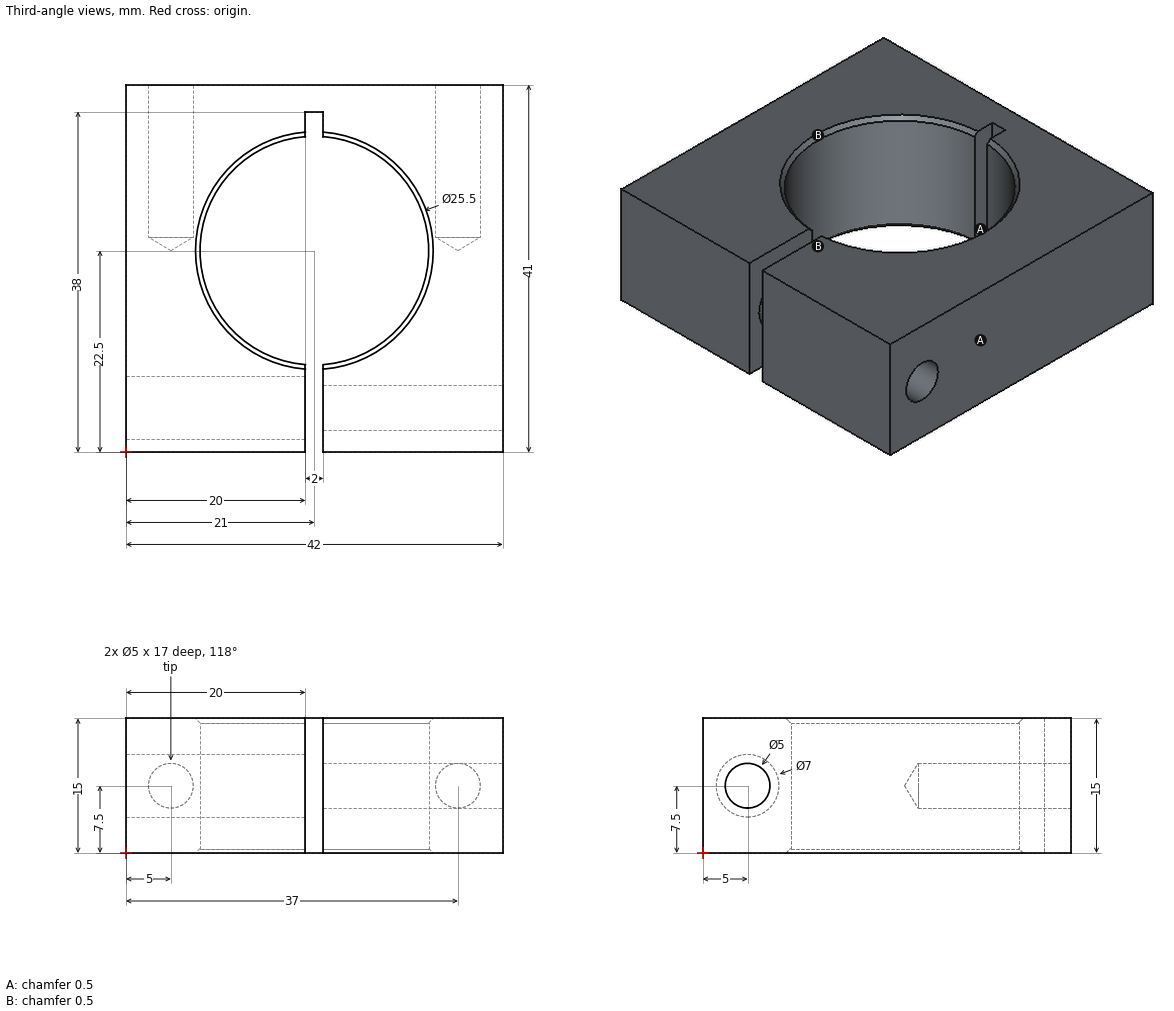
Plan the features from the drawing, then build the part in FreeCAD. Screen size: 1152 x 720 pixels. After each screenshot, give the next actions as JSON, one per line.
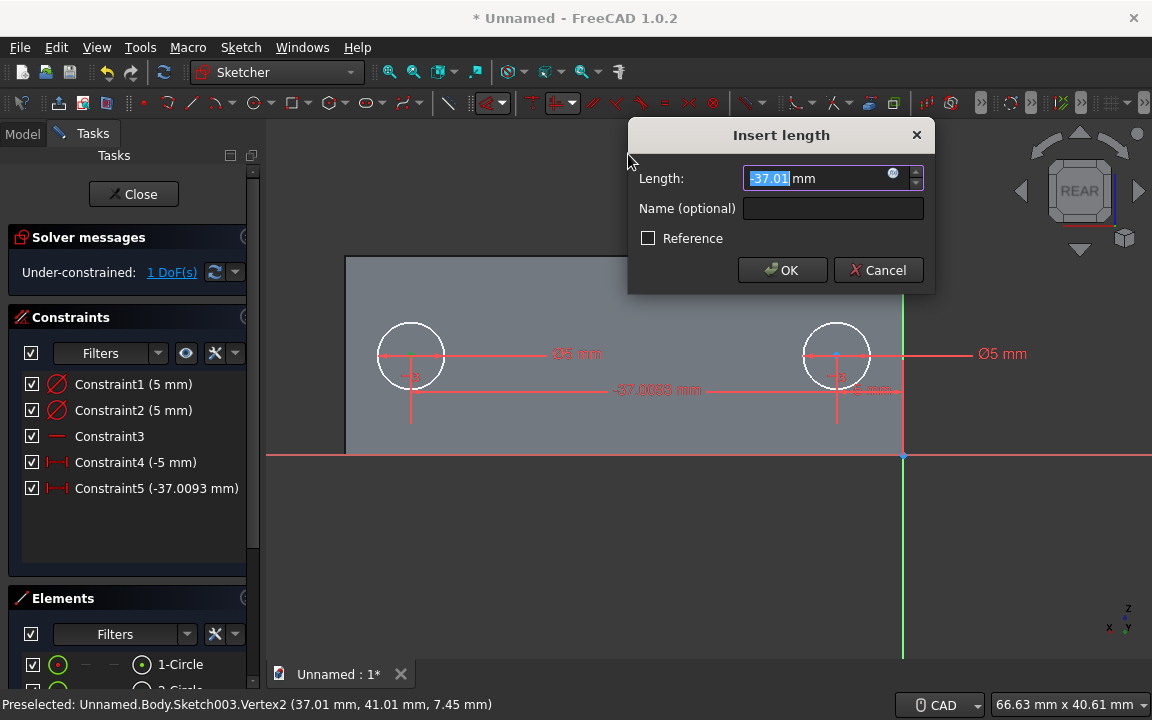
{"action": "type", "text": "-37"}
{"action": "key", "text": "Return"}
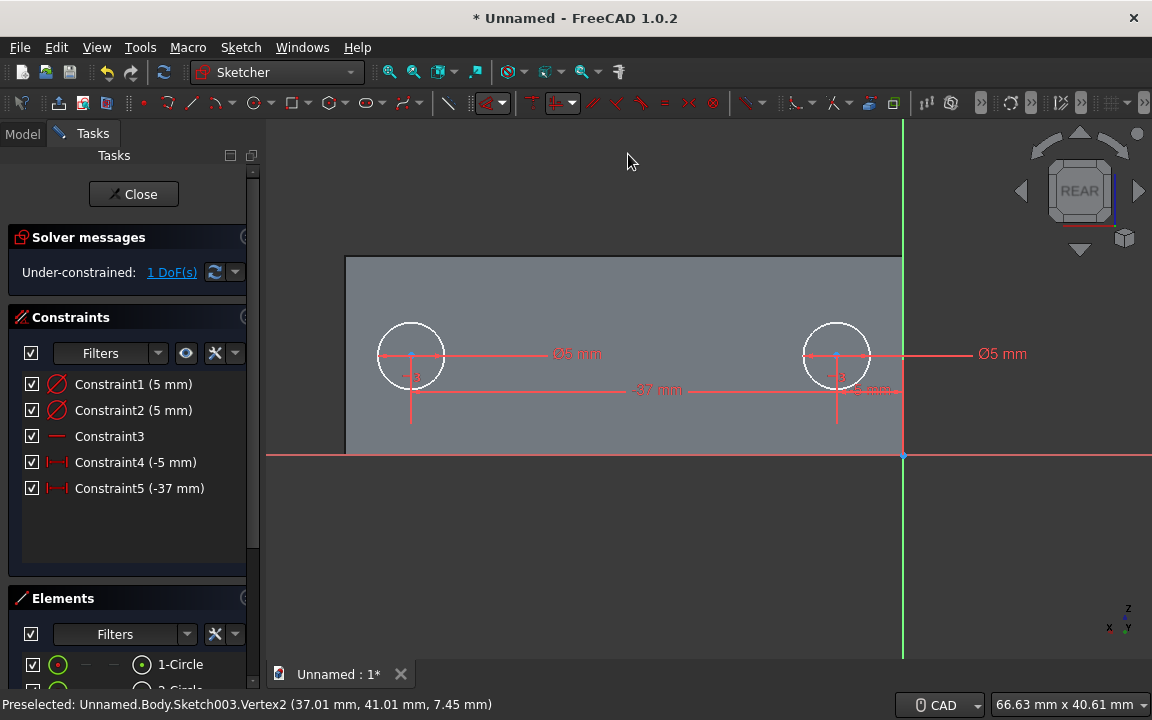
{"action": "left_click", "coordinate": [837, 356]}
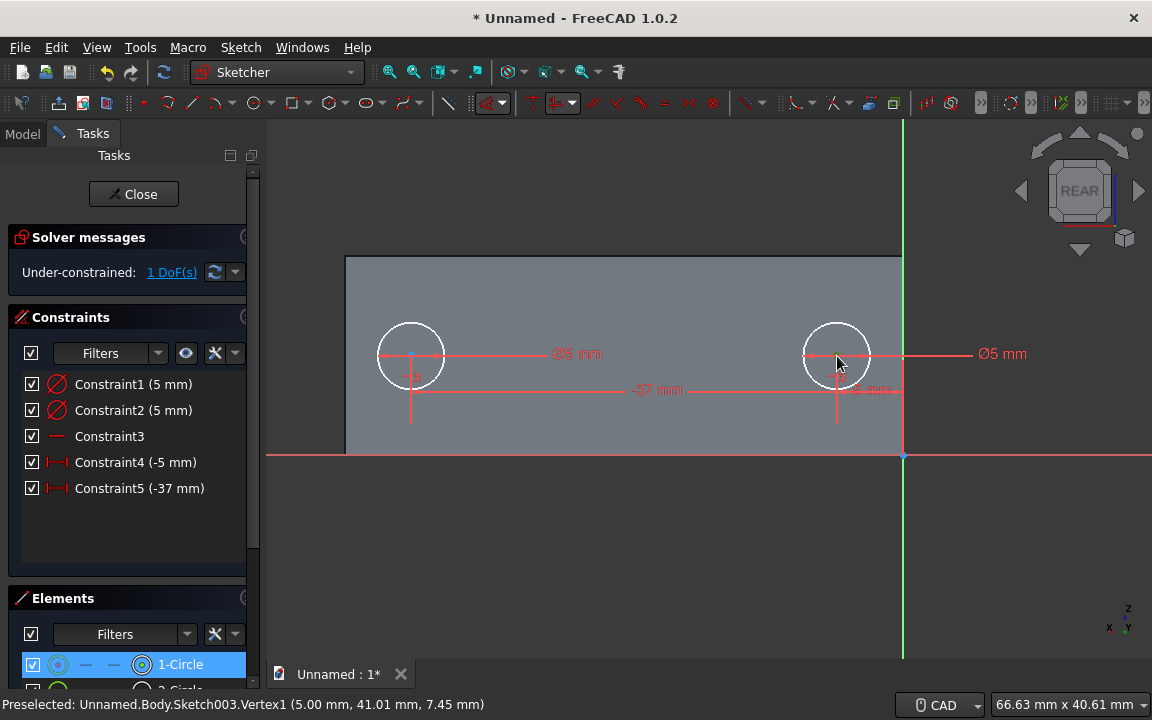
{"action": "left_click", "coordinate": [504, 104]}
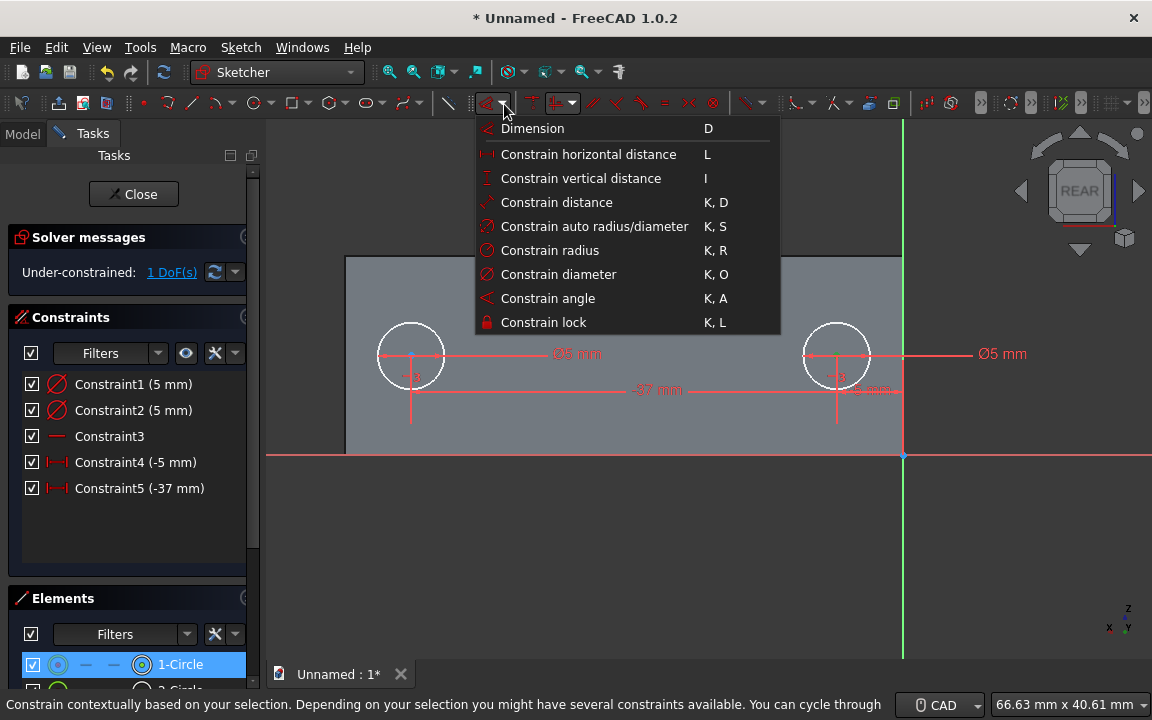
{"action": "left_click", "coordinate": [628, 178]}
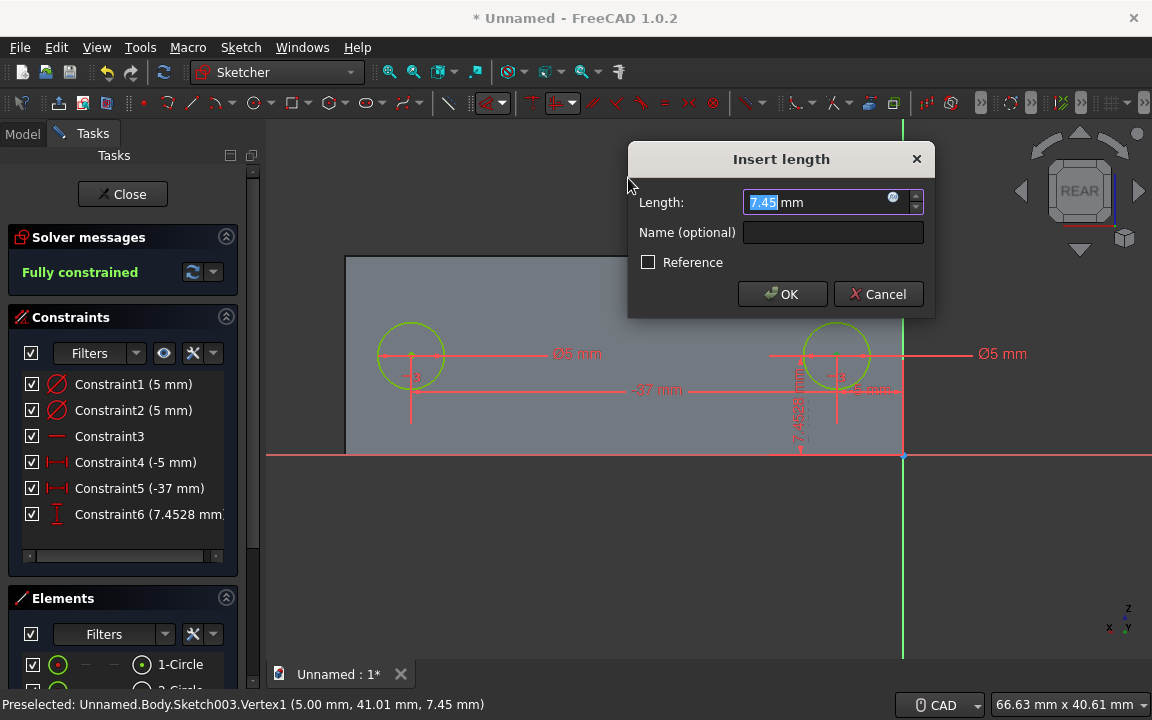
{"action": "type", "text": "7.5"}
{"action": "key", "text": "Return"}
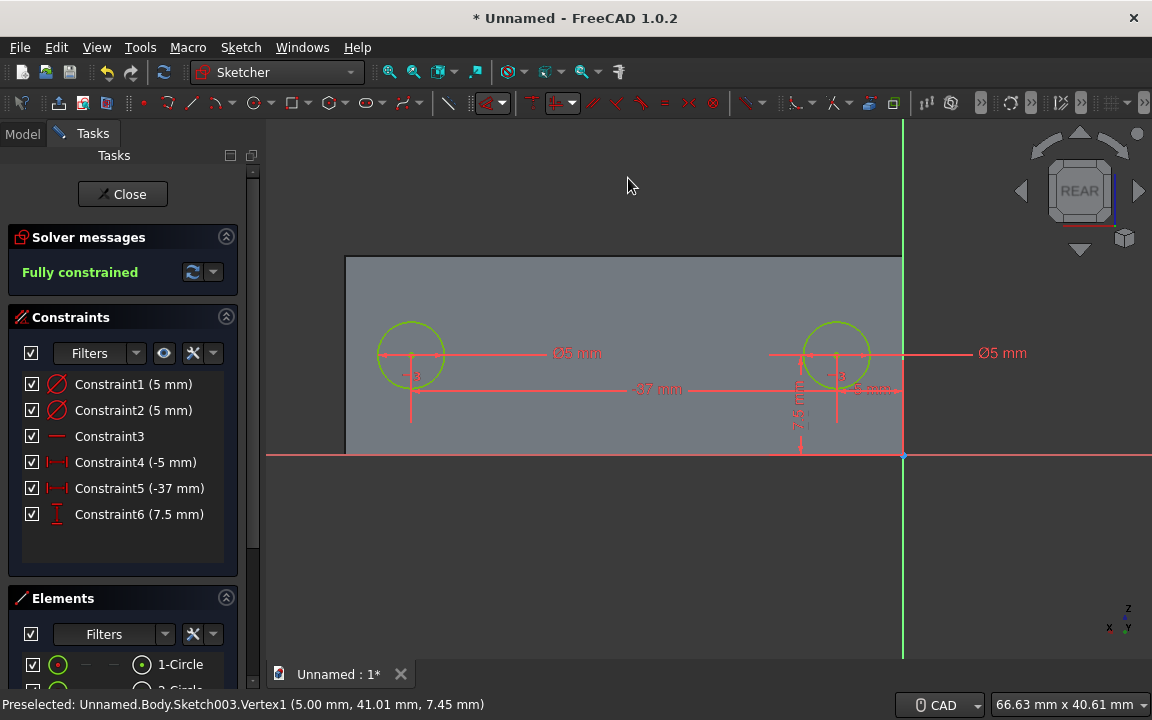
{"action": "left_click", "coordinate": [123, 194]}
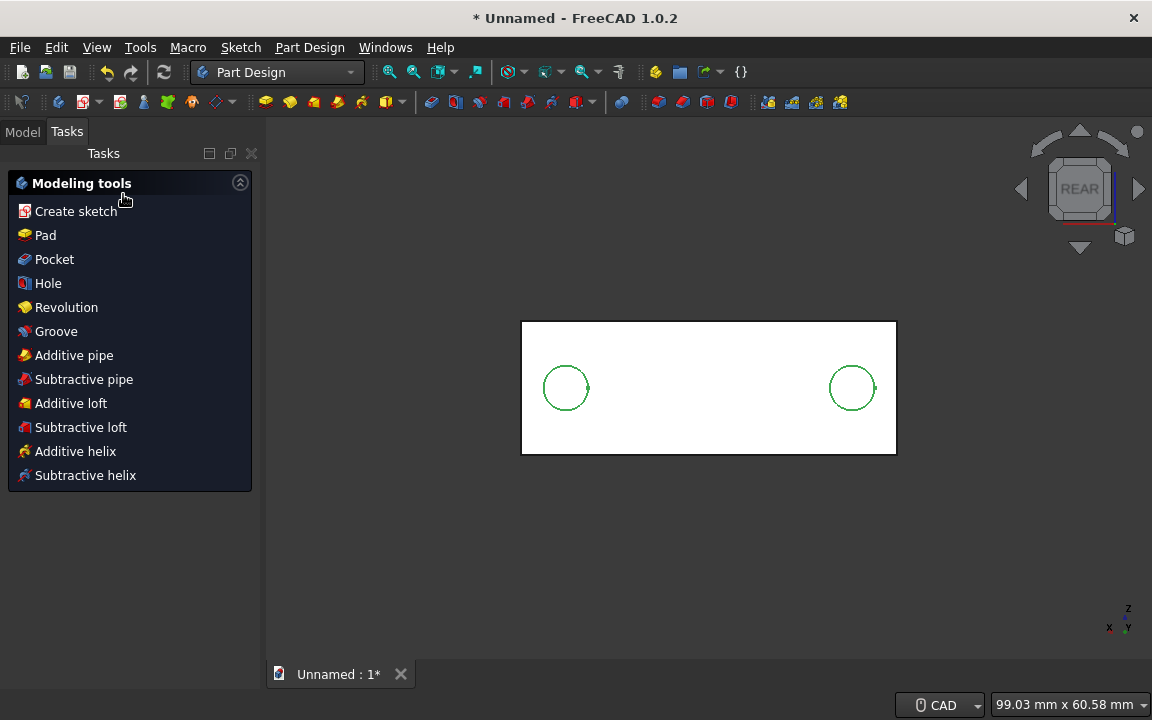
{"action": "left_click", "coordinate": [456, 102]}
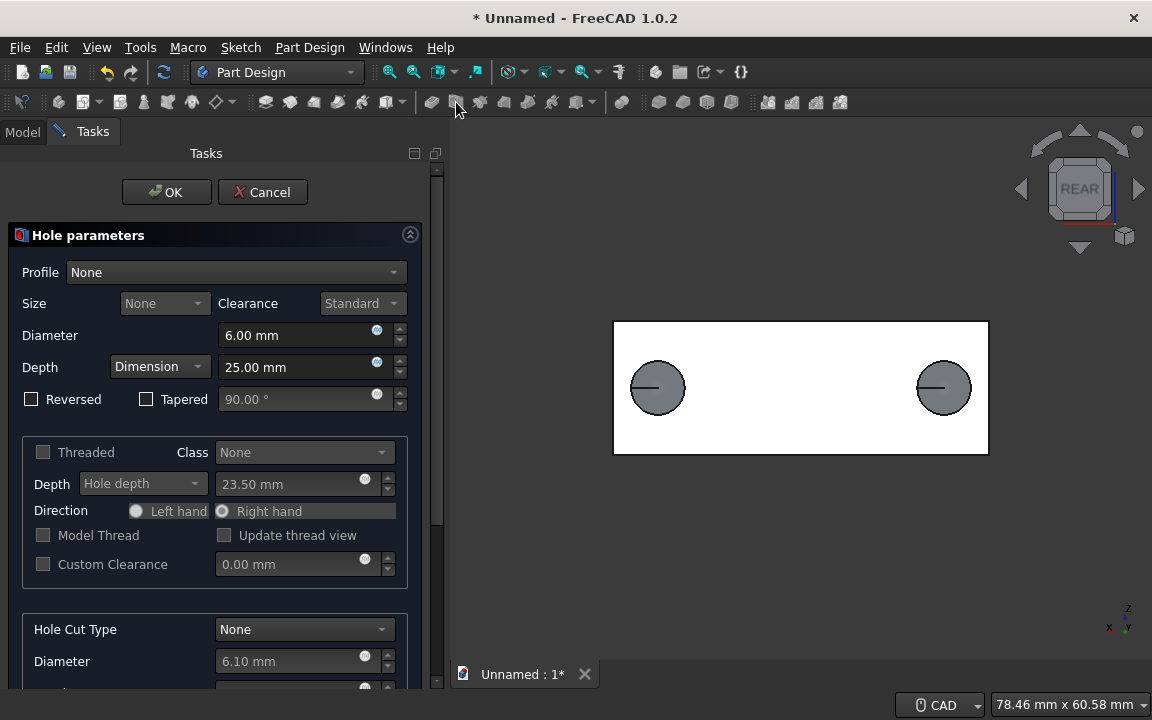
{"action": "triple_click", "coordinate": [305, 335]}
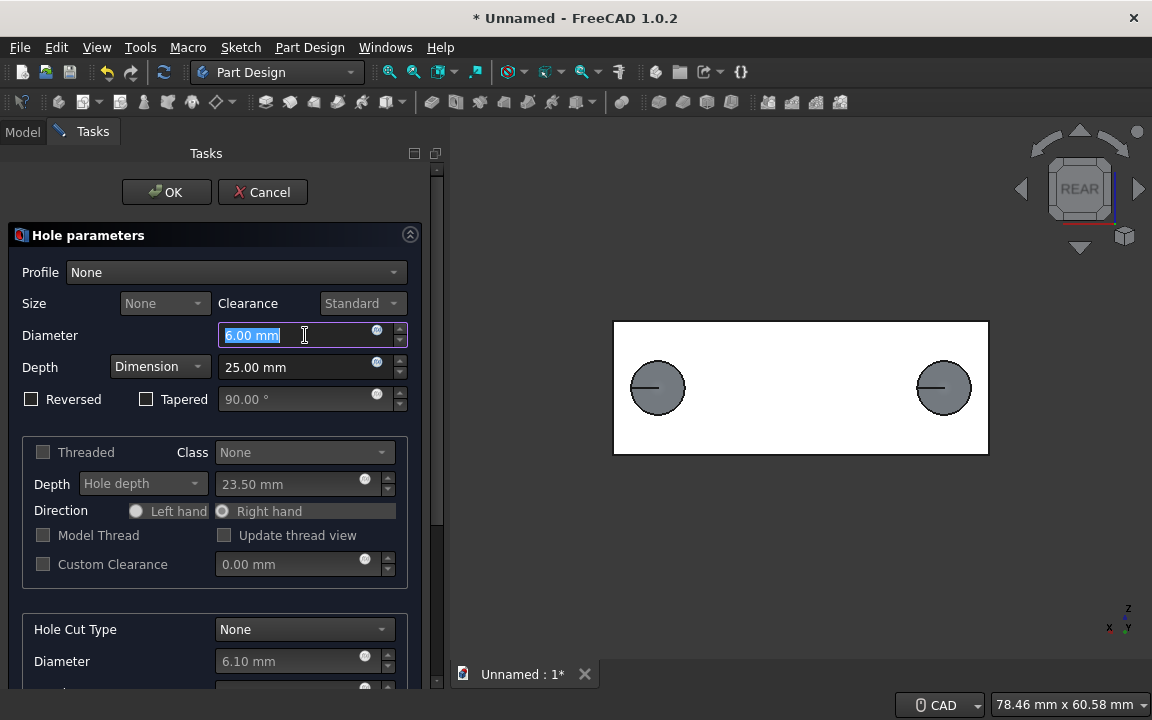
{"action": "type", "text": "5"}
{"action": "key", "text": "Tab"}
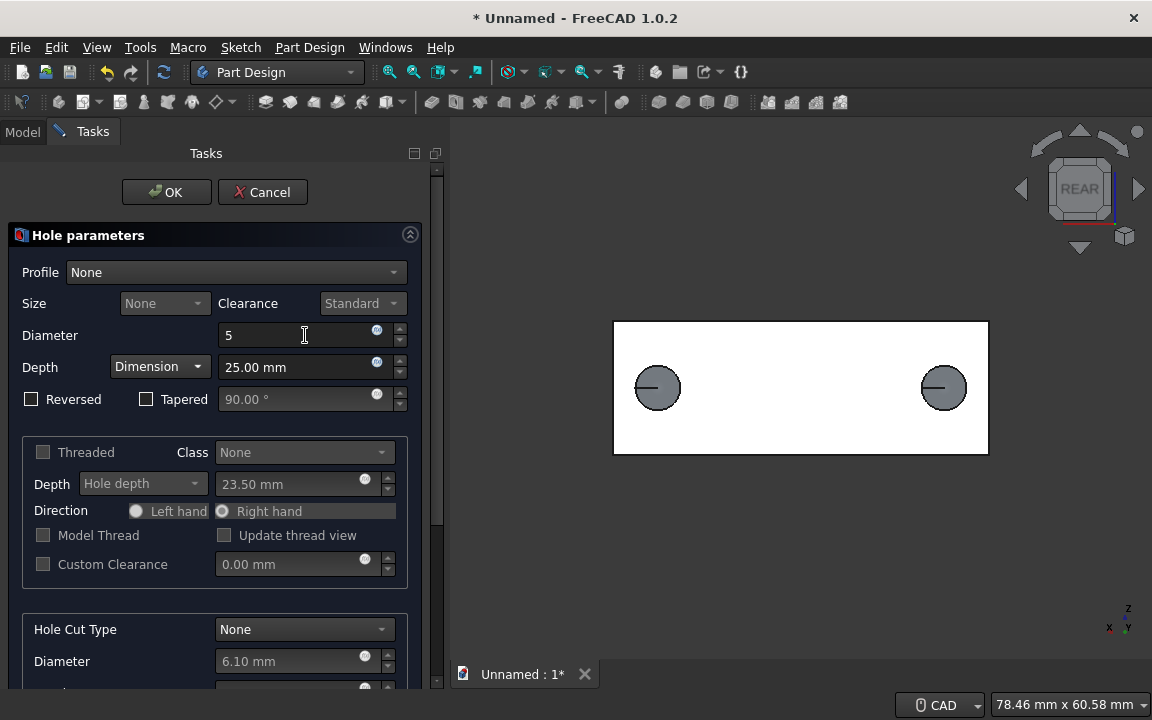
{"action": "triple_click", "coordinate": [305, 367]}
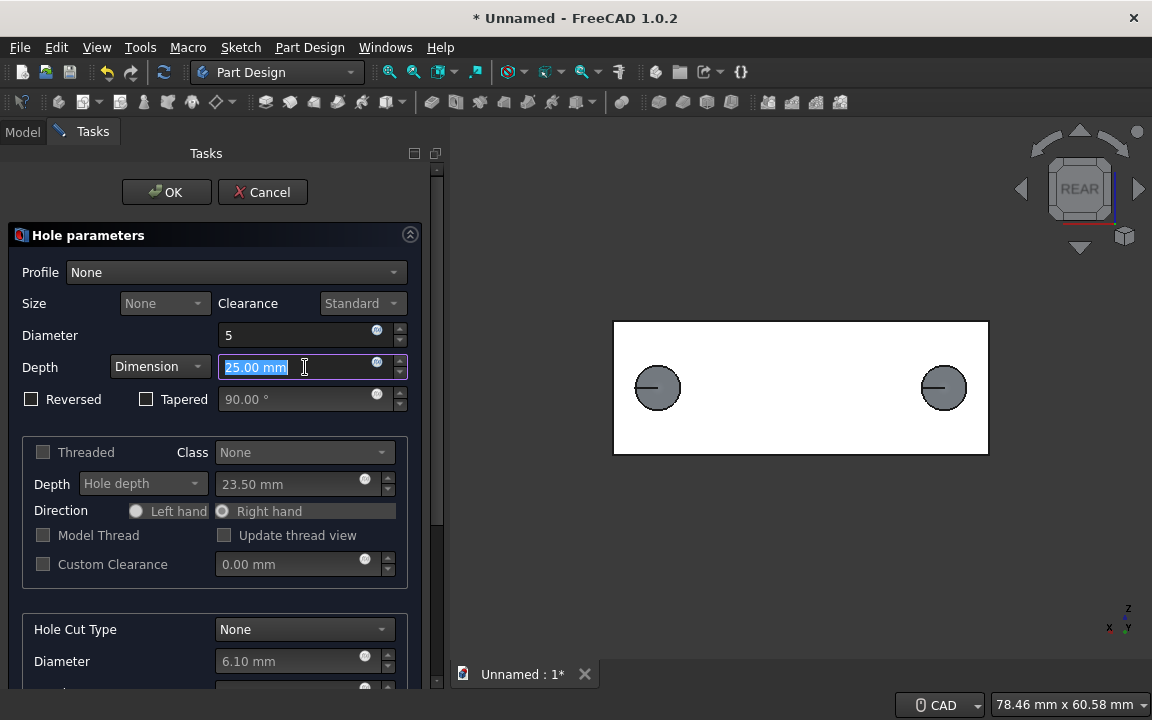
{"action": "type", "text": "17"}
{"action": "key", "text": "Tab"}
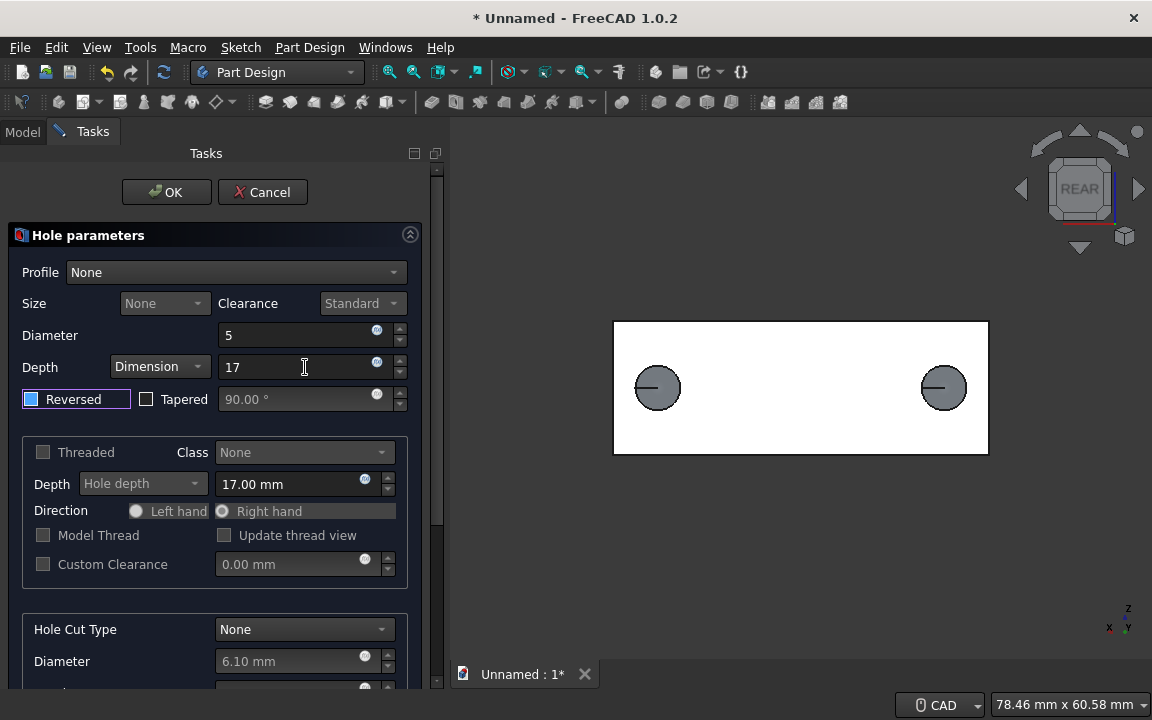
{"action": "left_click", "coordinate": [167, 192]}